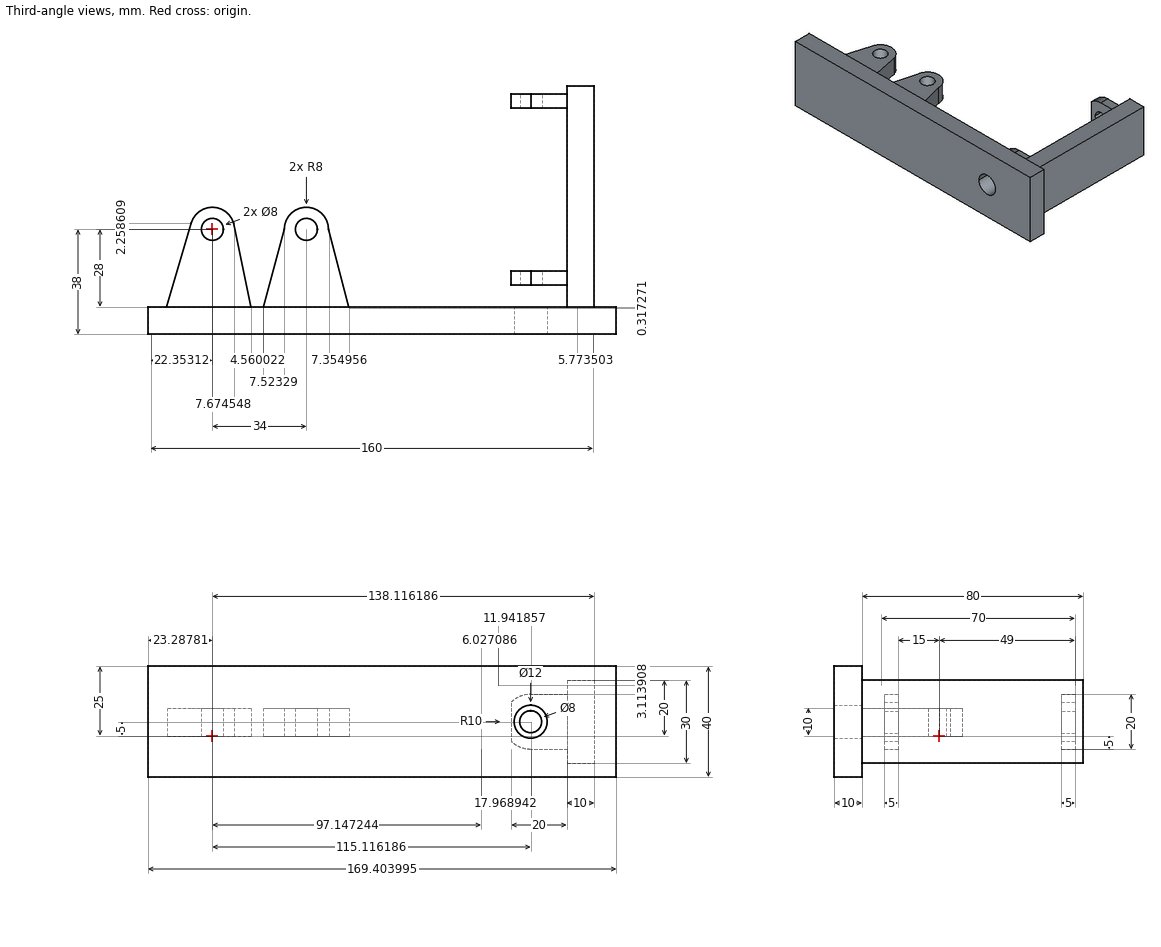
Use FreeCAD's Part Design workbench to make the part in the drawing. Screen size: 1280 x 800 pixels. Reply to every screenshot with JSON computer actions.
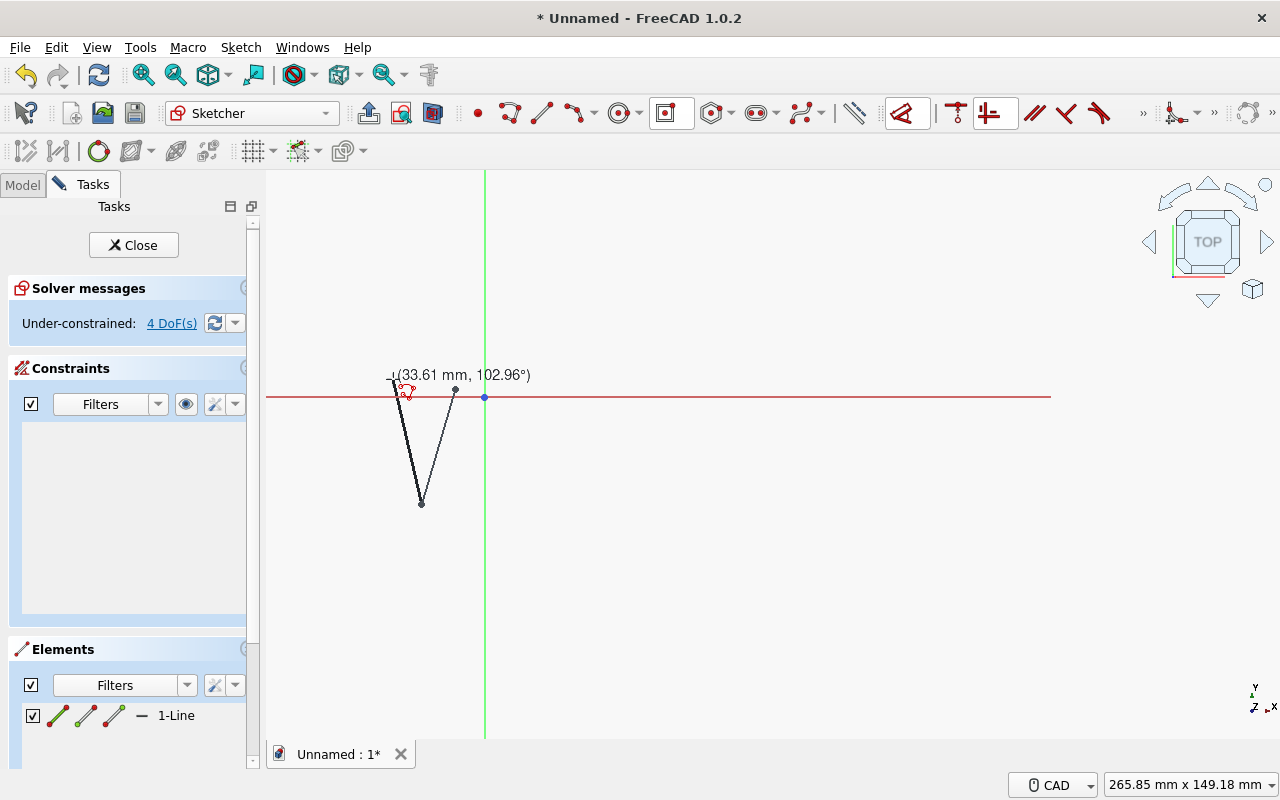
{"action": "left_click", "coordinate": [400, 542]}
{"action": "left_click", "coordinate": [1010, 542]}
{"action": "left_click", "coordinate": [988, 504]}
{"action": "left_click", "coordinate": [673, 520]}
{"action": "left_click", "coordinate": [645, 397]}
{"action": "right_click", "coordinate": [645, 397]}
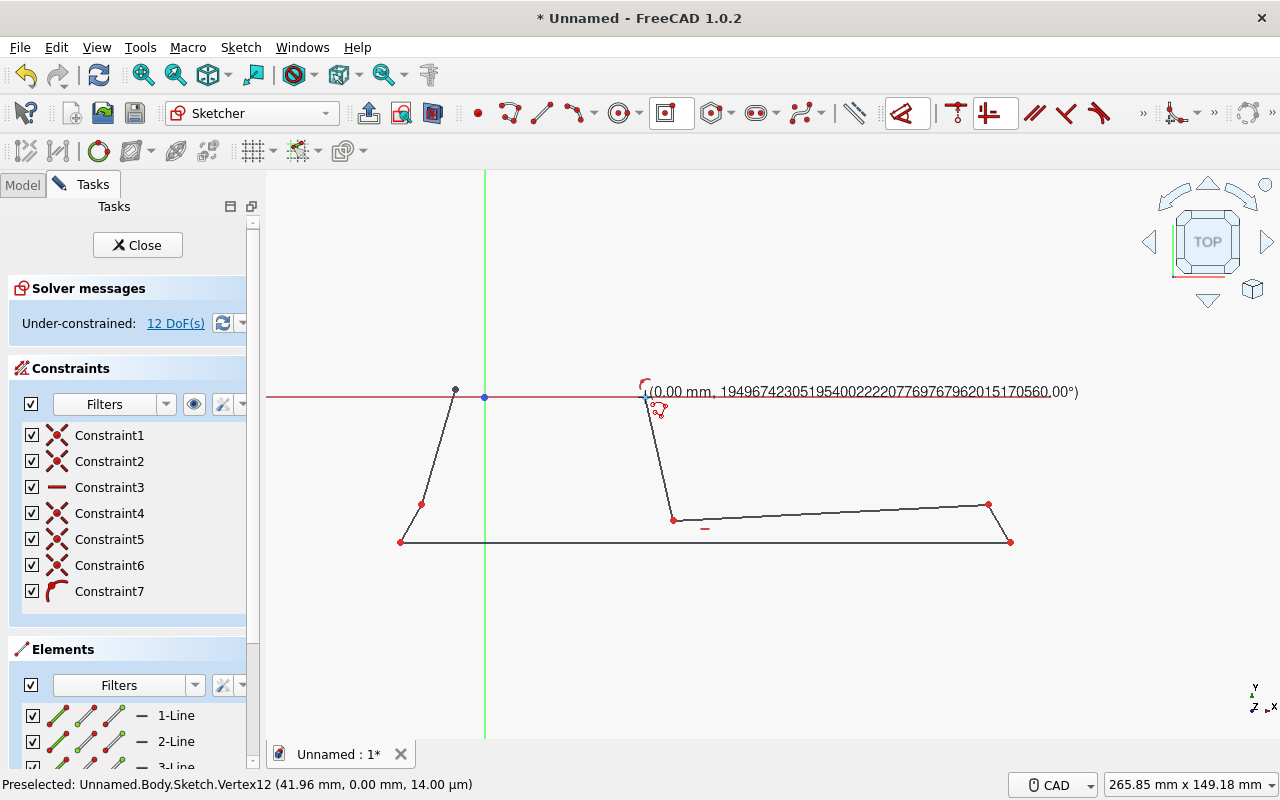
{"action": "left_click", "coordinate": [584, 397]}
{"action": "left_click", "coordinate": [555, 504]}
{"action": "left_click", "coordinate": [538, 504]}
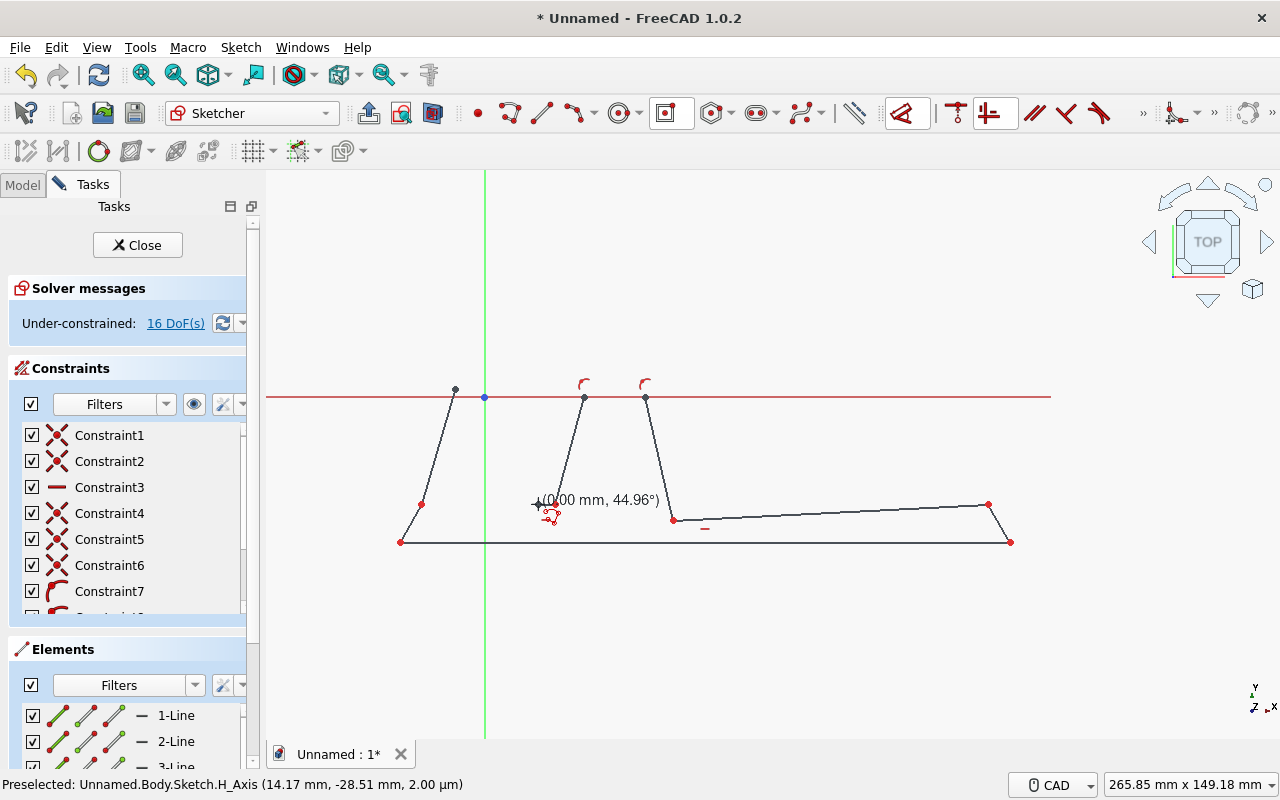
{"action": "scroll", "coordinate": [514, 389], "scroll_direction": "up", "scroll_amount": 4}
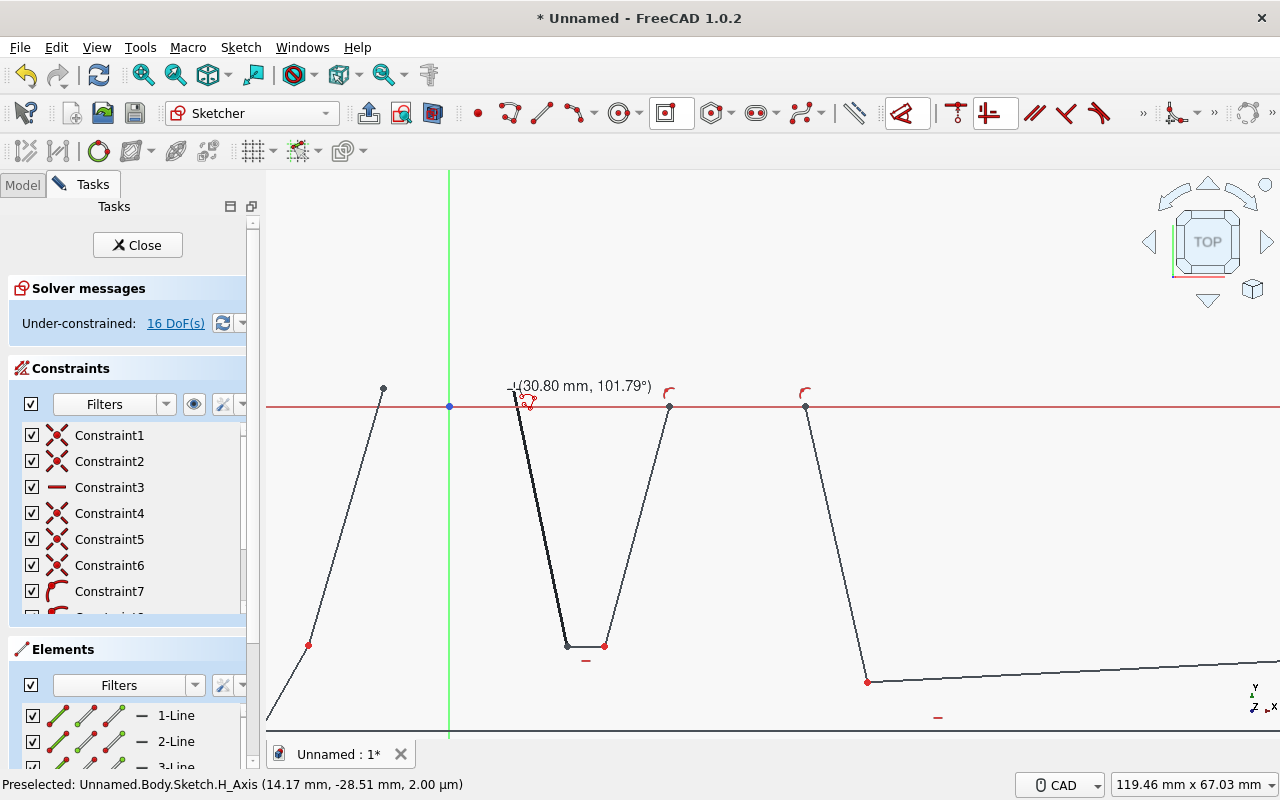
{"action": "left_click", "coordinate": [514, 388]}
{"action": "right_click", "coordinate": [514, 388]}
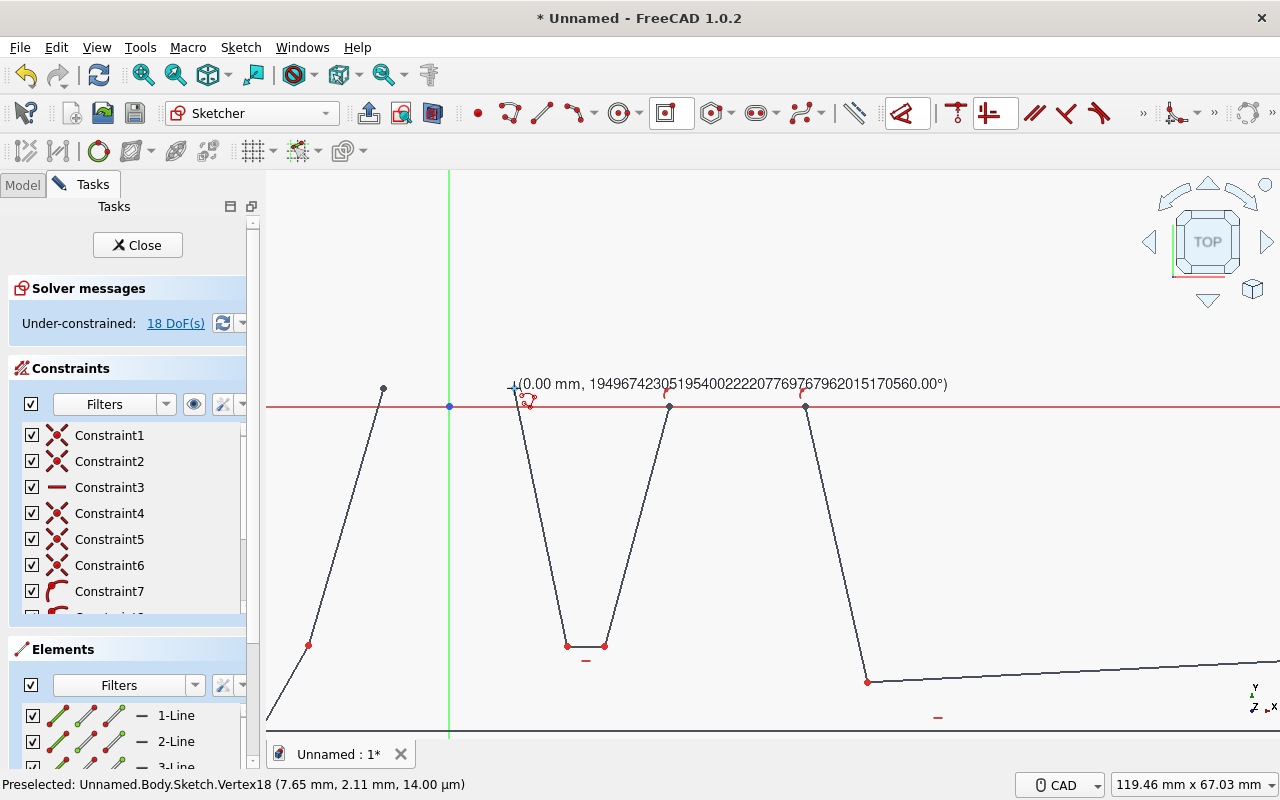
{"action": "left_click", "coordinate": [574, 114]}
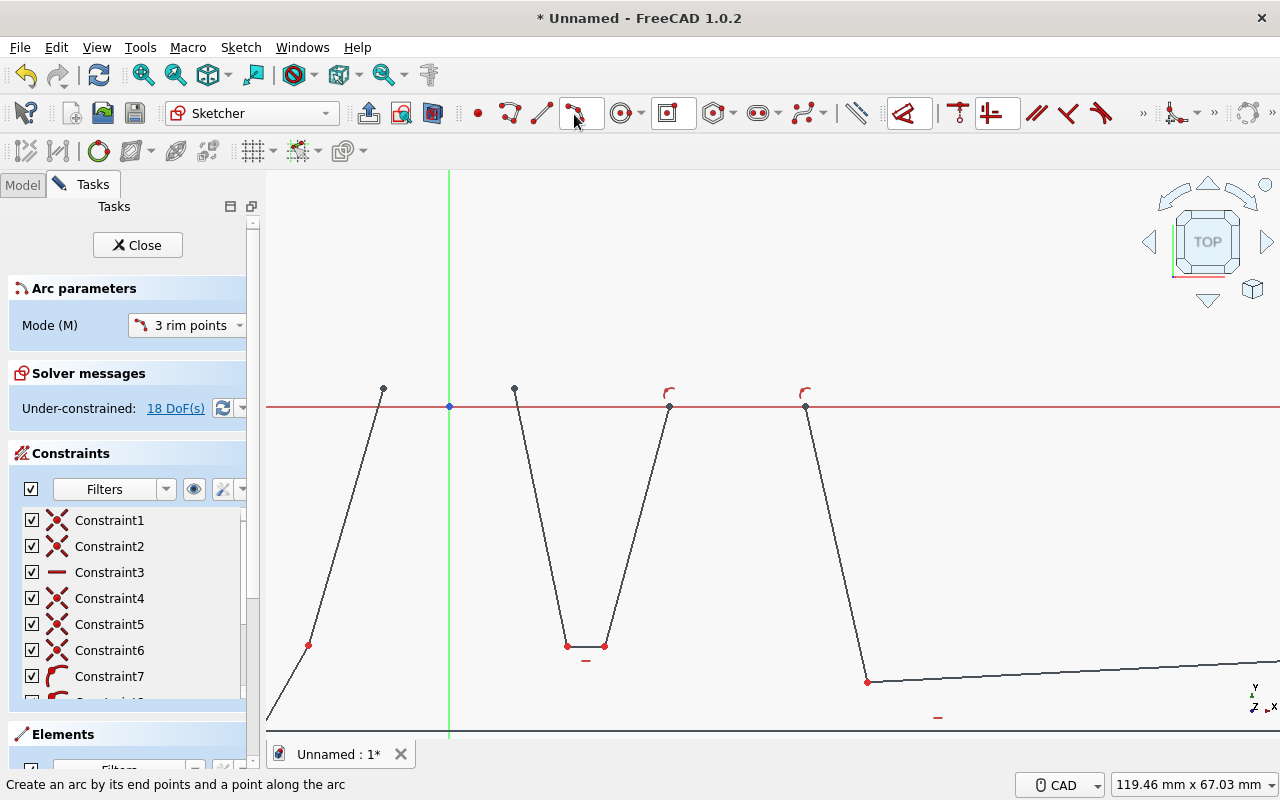
{"action": "left_click", "coordinate": [805, 407]}
{"action": "left_click", "coordinate": [669, 407]}
{"action": "left_click", "coordinate": [738, 339]}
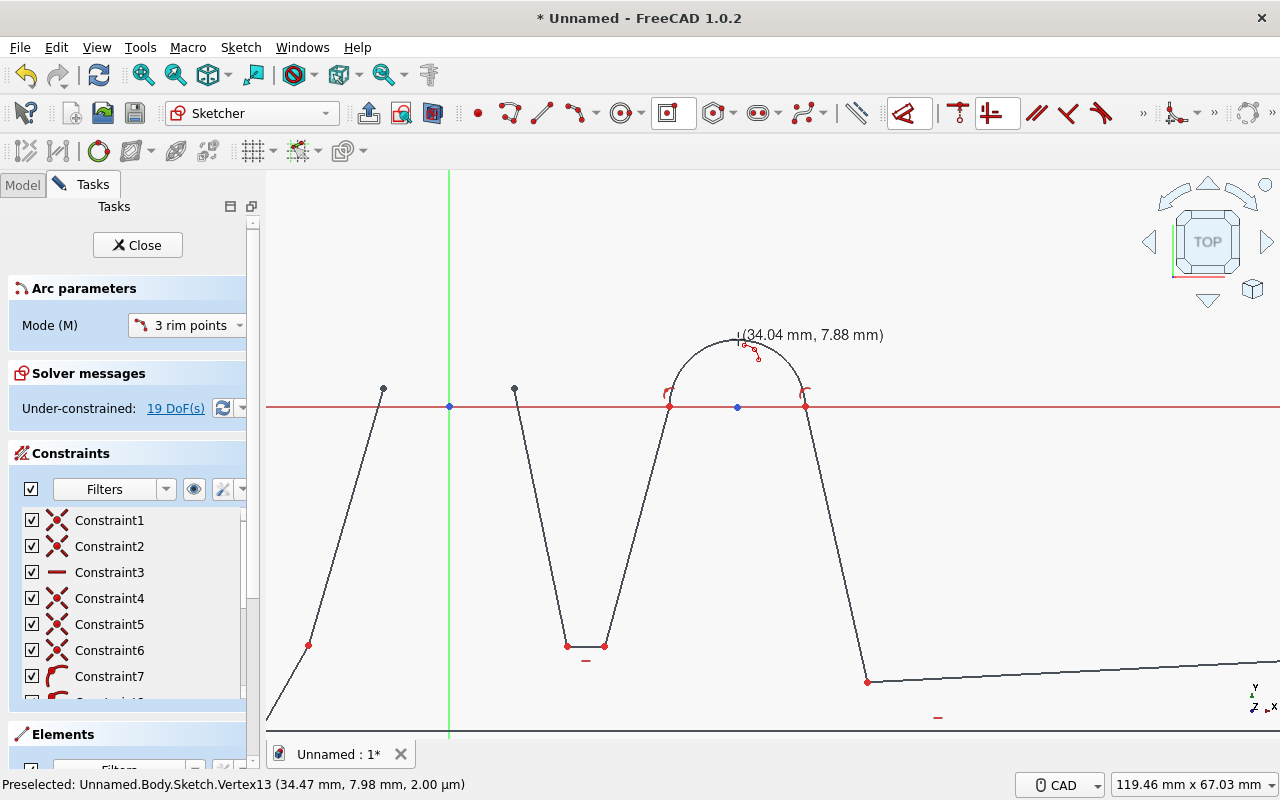
{"action": "left_click", "coordinate": [514, 389]}
{"action": "left_click", "coordinate": [384, 389]}
{"action": "left_click", "coordinate": [416, 348]}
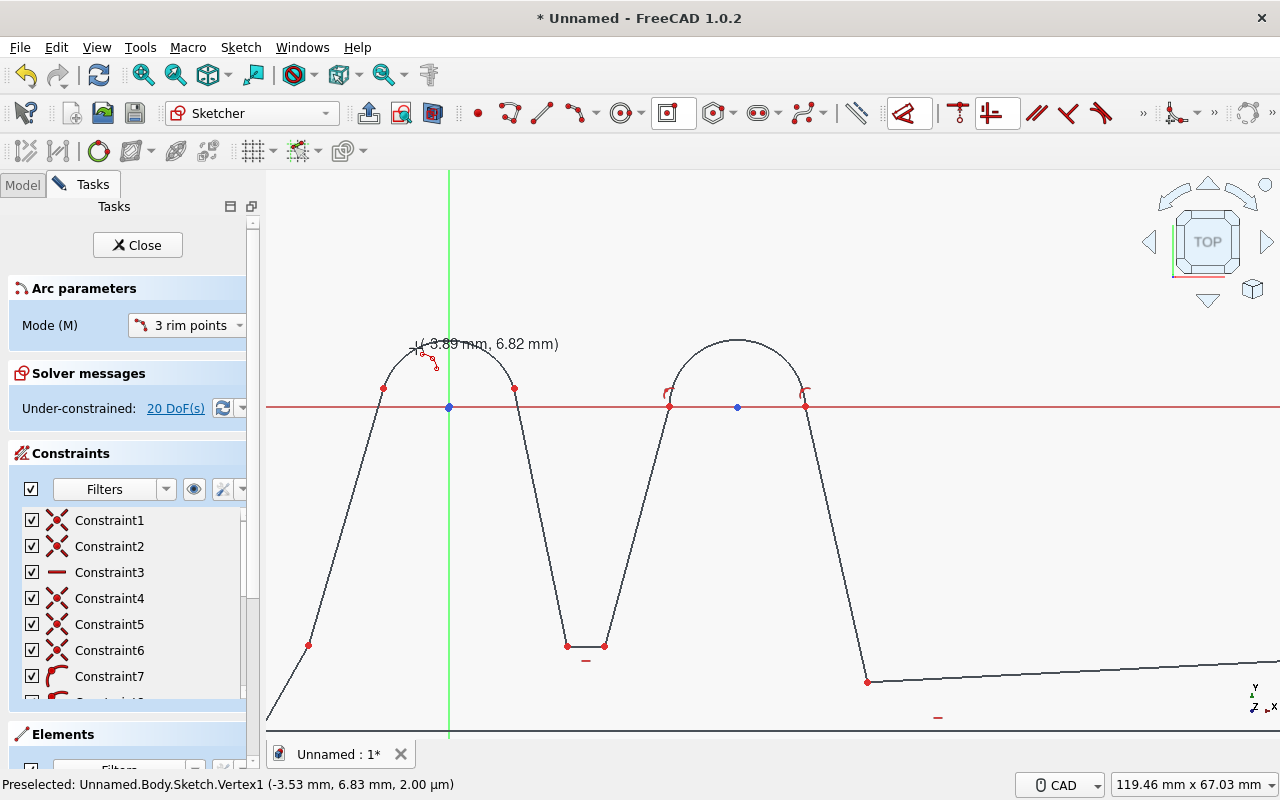
{"action": "left_click", "coordinate": [622, 114]}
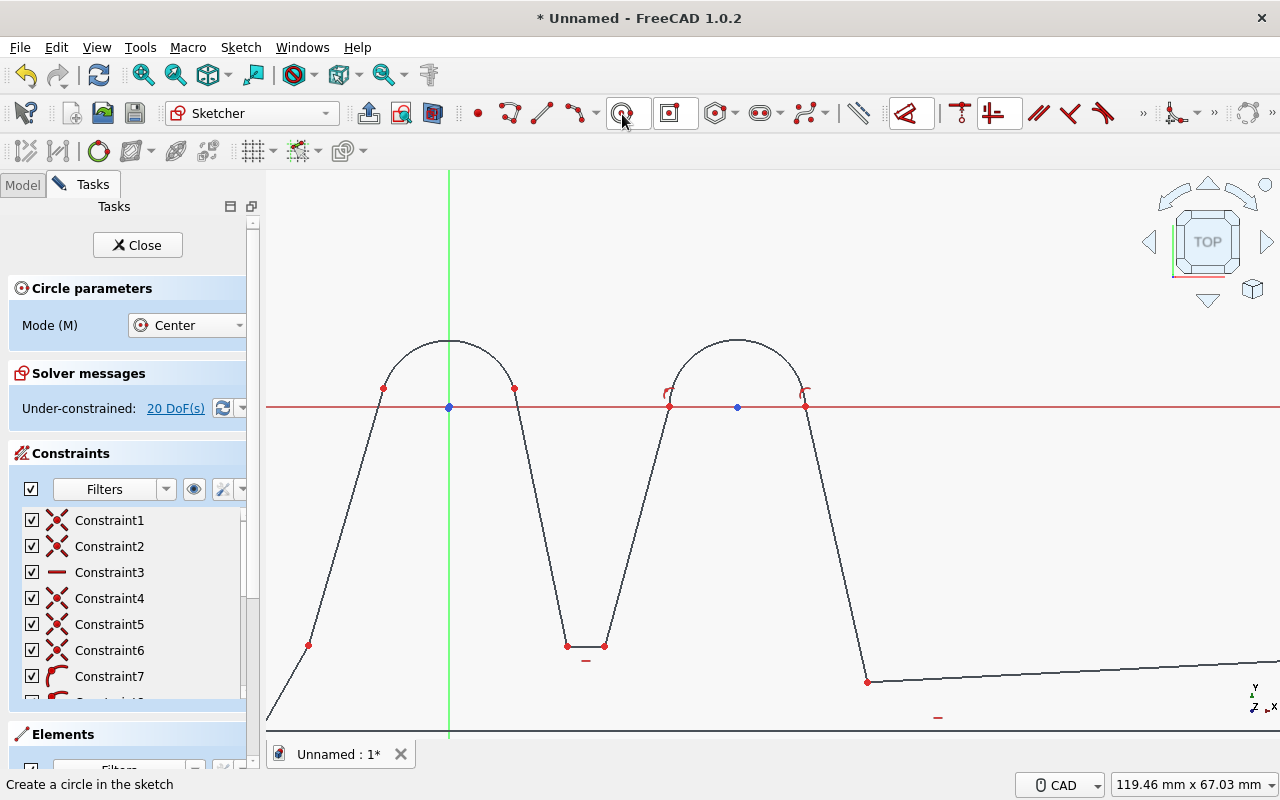
{"action": "left_click", "coordinate": [449, 407]}
{"action": "mouse_move", "coordinate": [473, 383]}